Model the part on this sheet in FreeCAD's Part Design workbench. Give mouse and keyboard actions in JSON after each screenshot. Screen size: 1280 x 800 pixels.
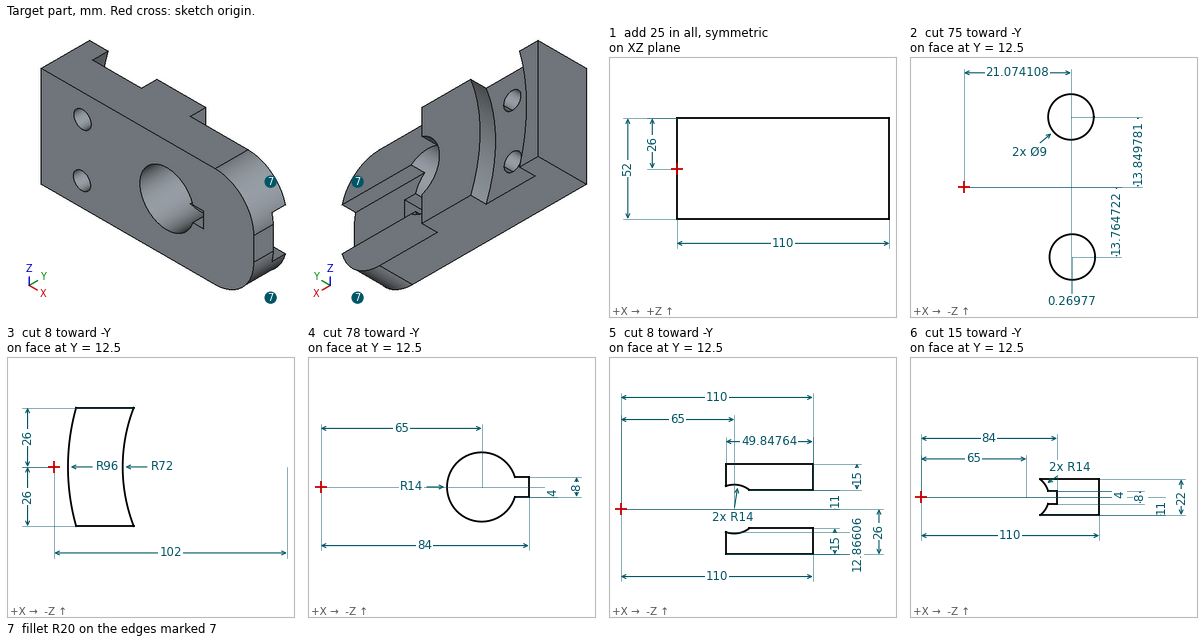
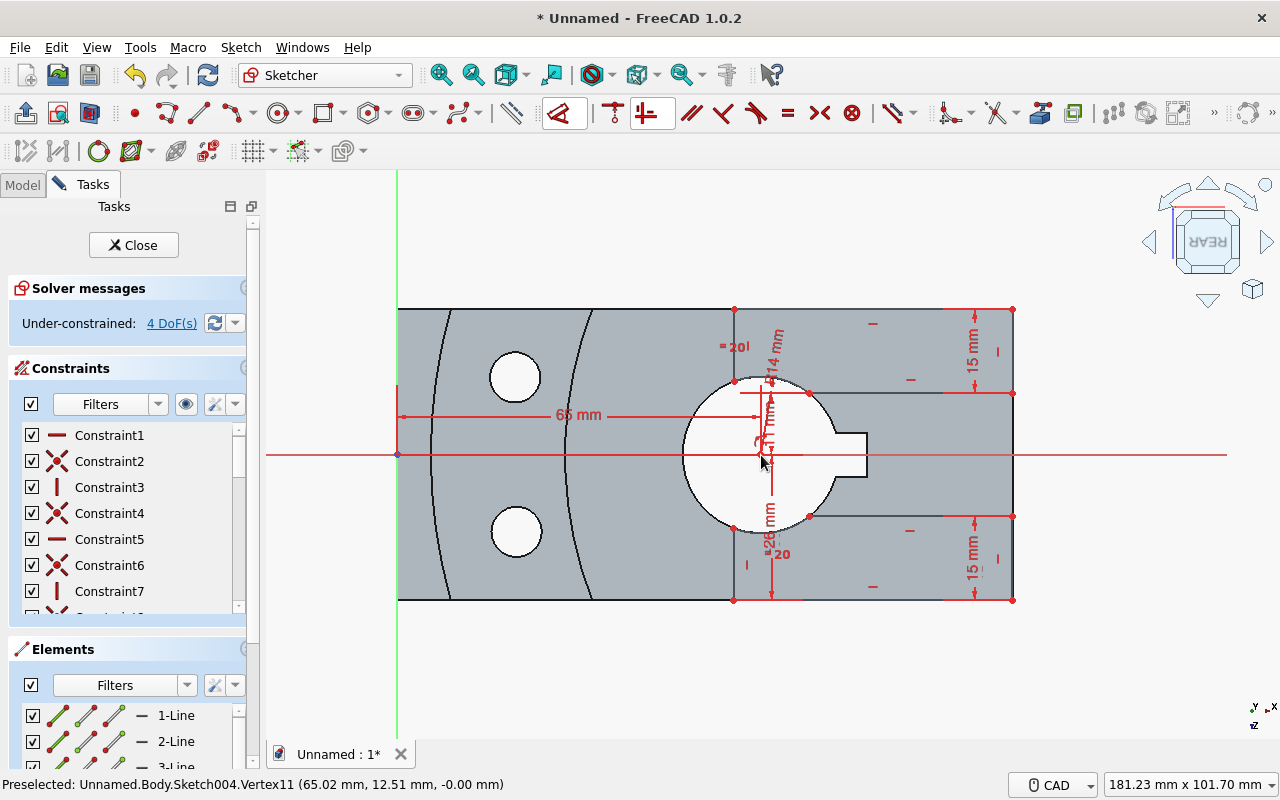
{"action": "left_click", "coordinate": [1013, 393]}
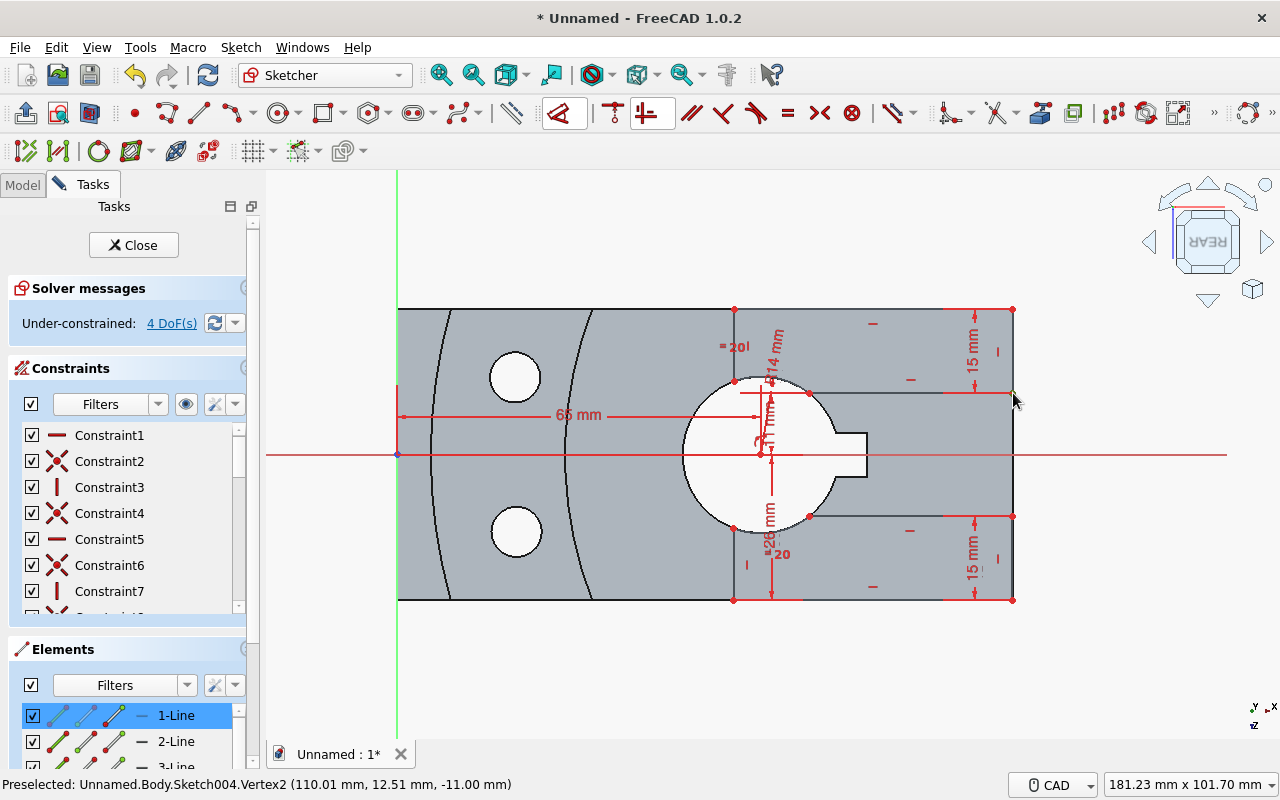
{"action": "left_click", "coordinate": [582, 114]}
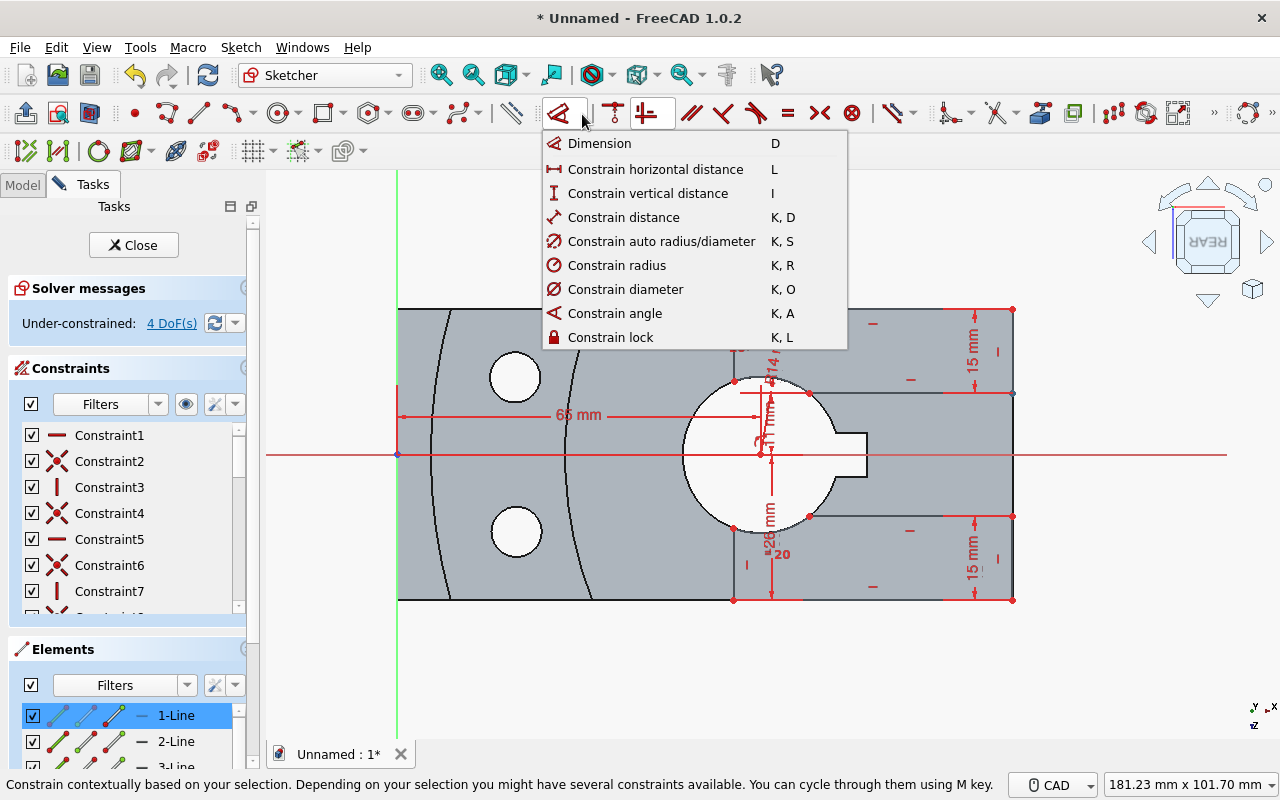
{"action": "left_click", "coordinate": [695, 169]}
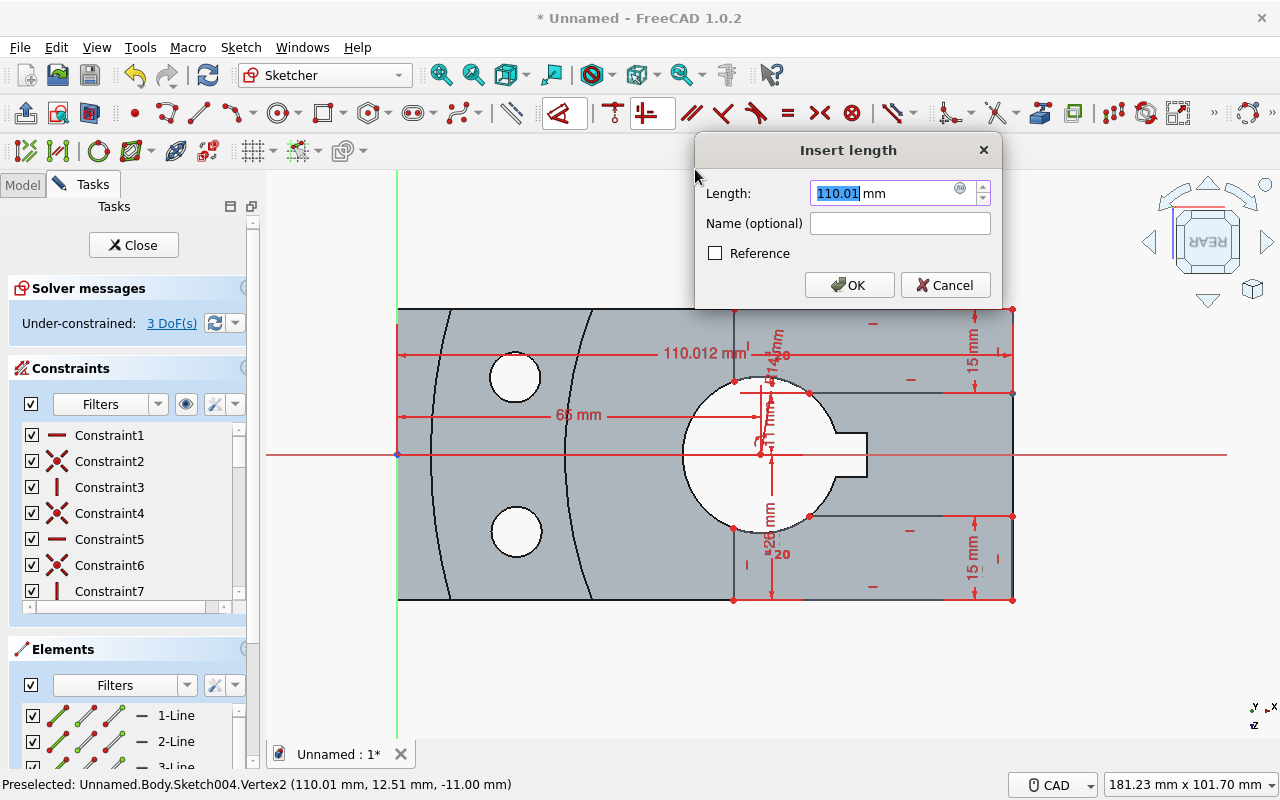
{"action": "type", "text": "110"}
{"action": "key", "text": "Return"}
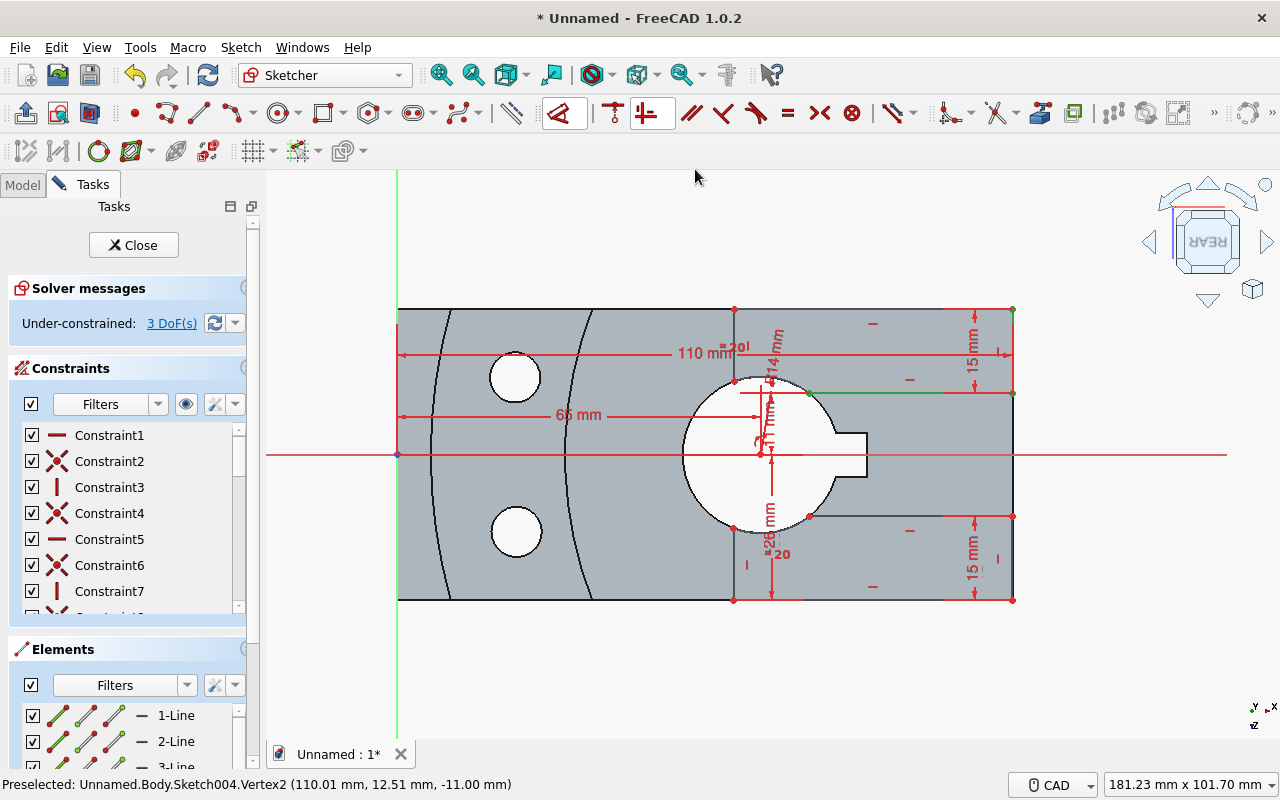
{"action": "left_click", "coordinate": [1012, 600]}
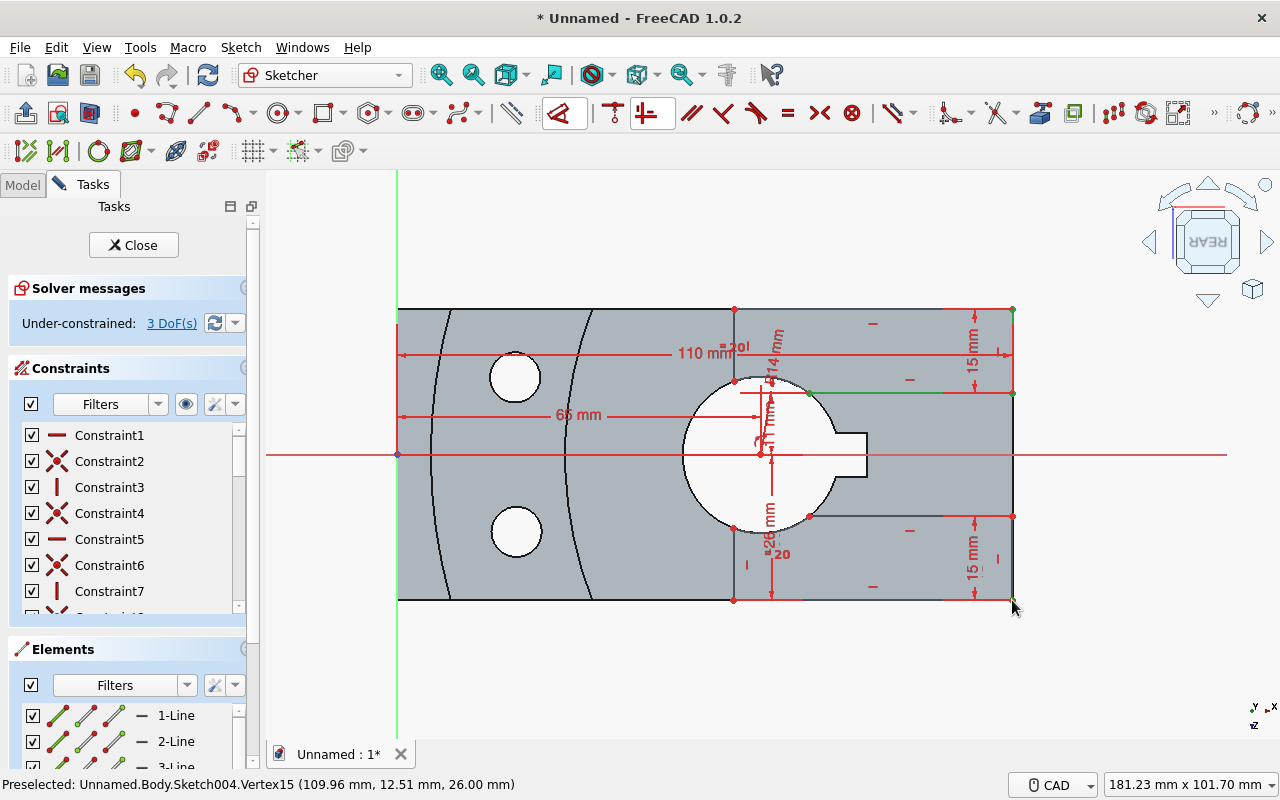
{"action": "left_click", "coordinate": [582, 114]}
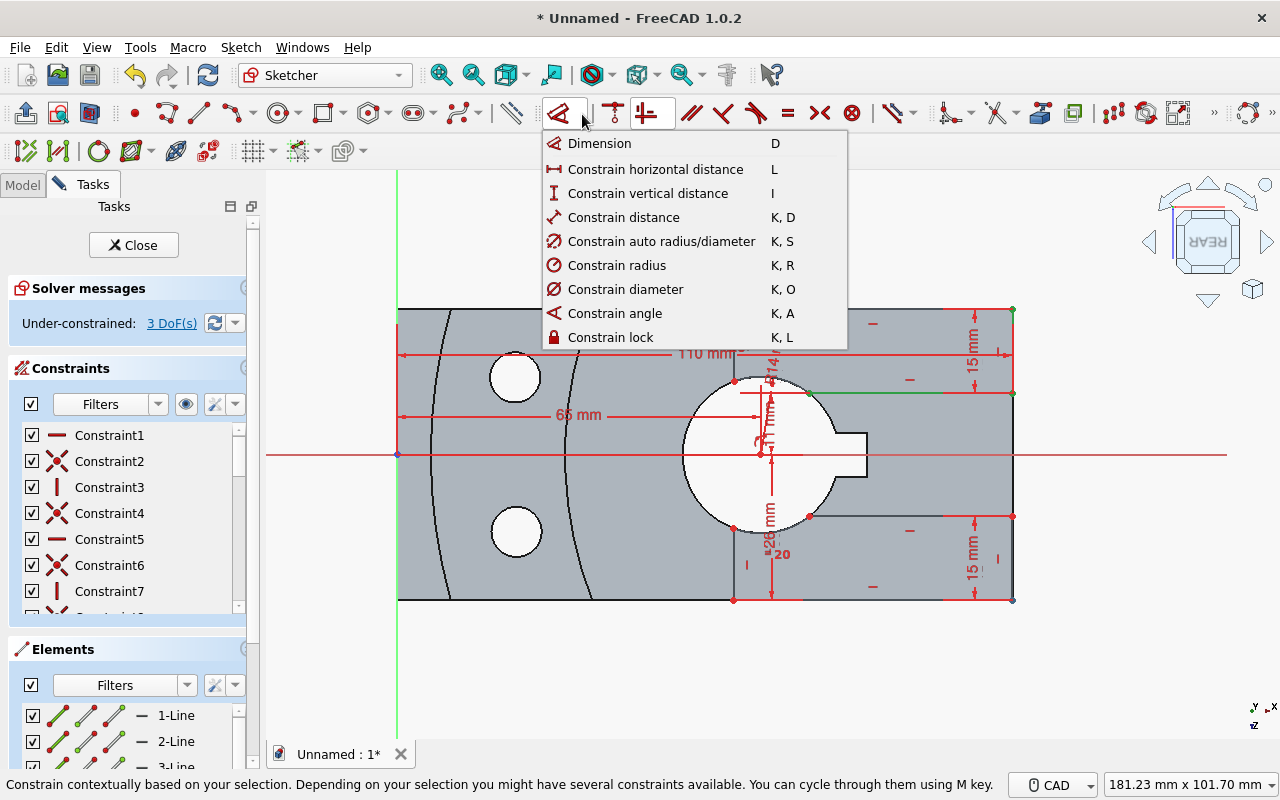
{"action": "left_click", "coordinate": [695, 169]}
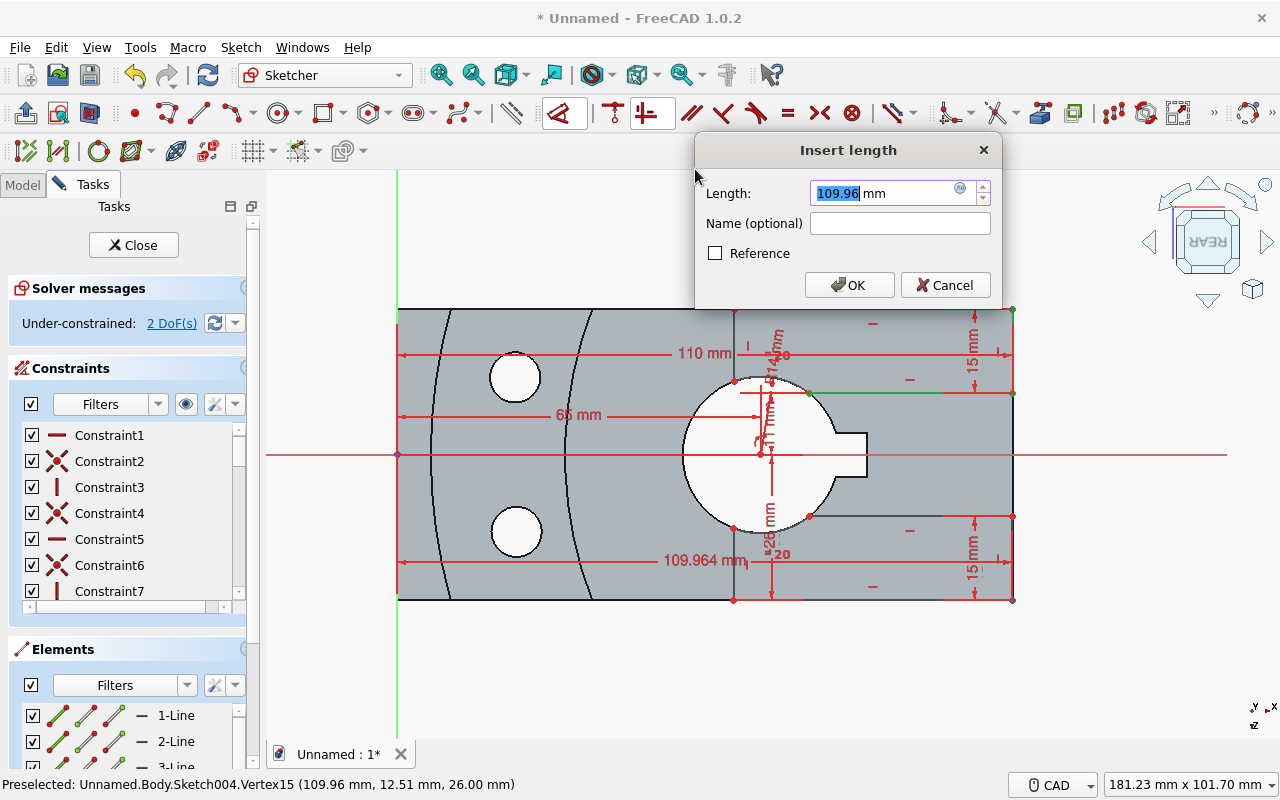
{"action": "type", "text": "110"}
{"action": "key", "text": "Return"}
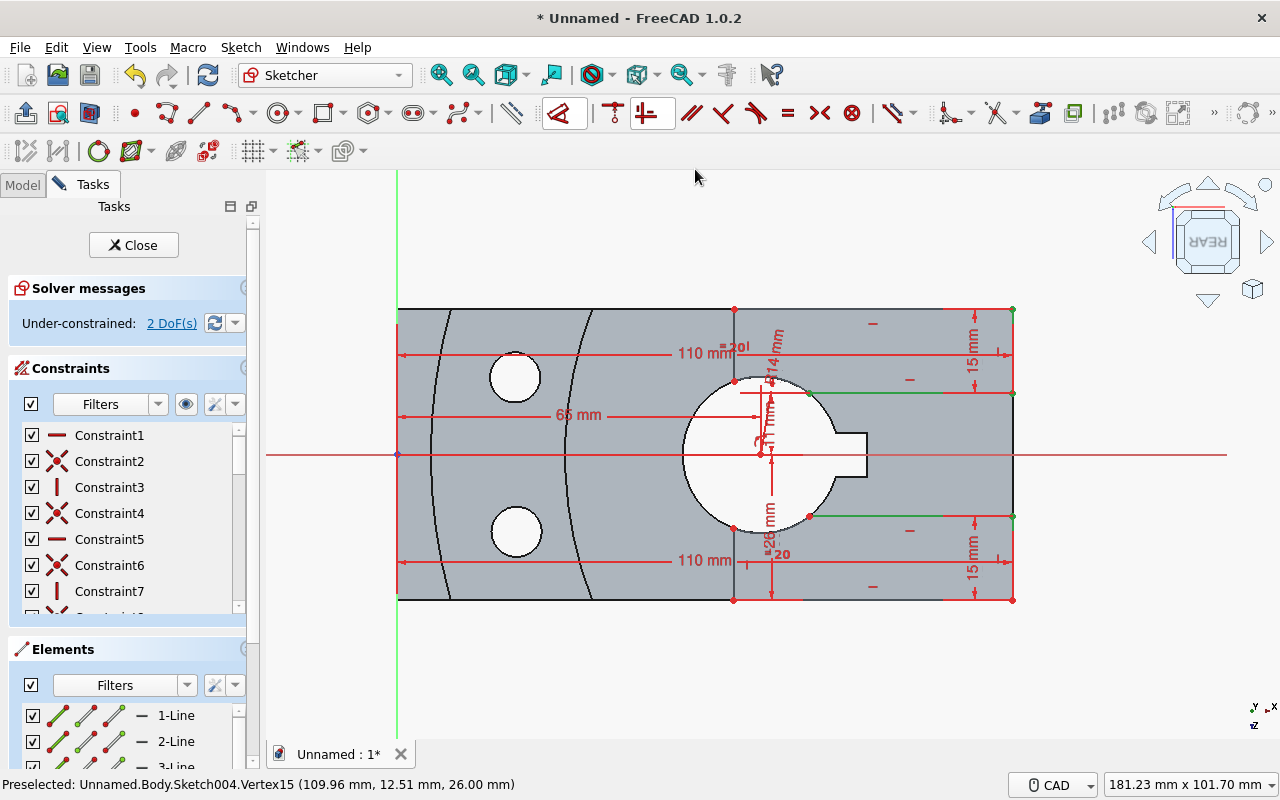
{"action": "left_click", "coordinate": [929, 309]}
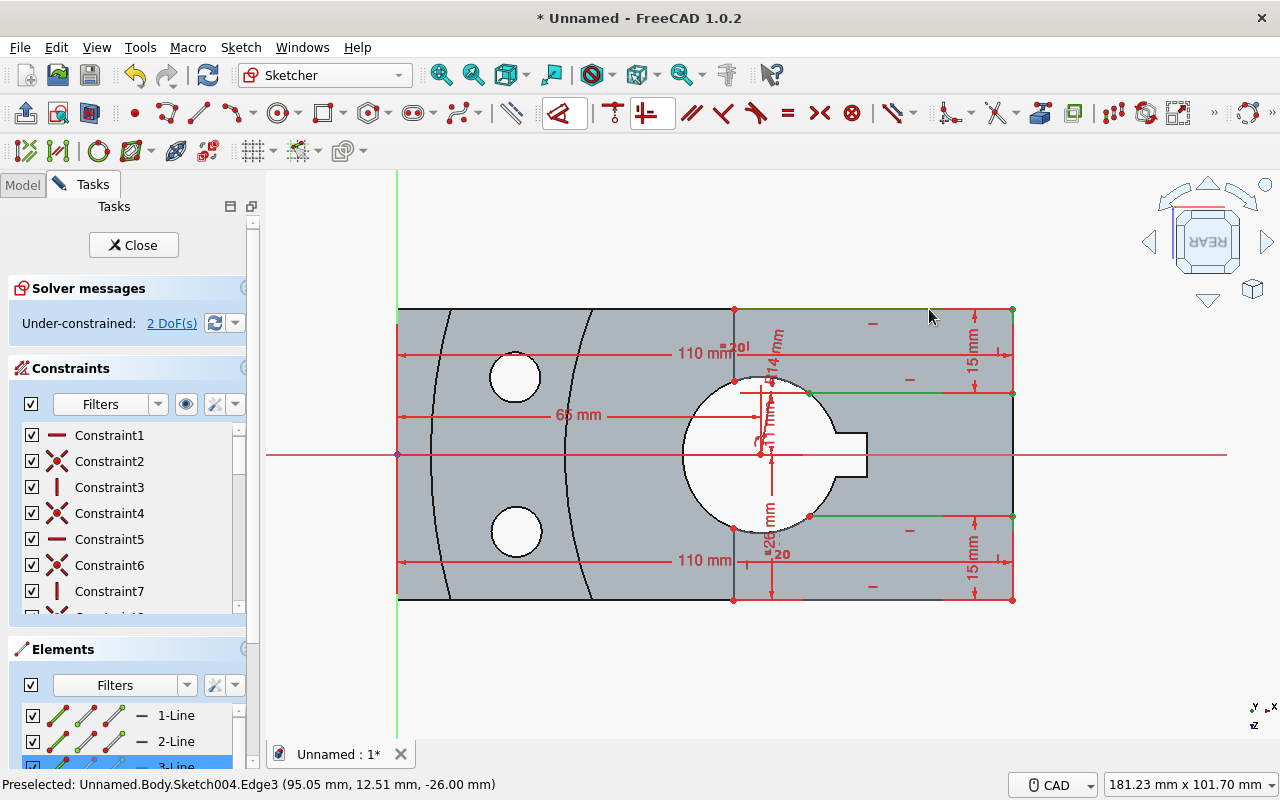
{"action": "left_click", "coordinate": [582, 114]}